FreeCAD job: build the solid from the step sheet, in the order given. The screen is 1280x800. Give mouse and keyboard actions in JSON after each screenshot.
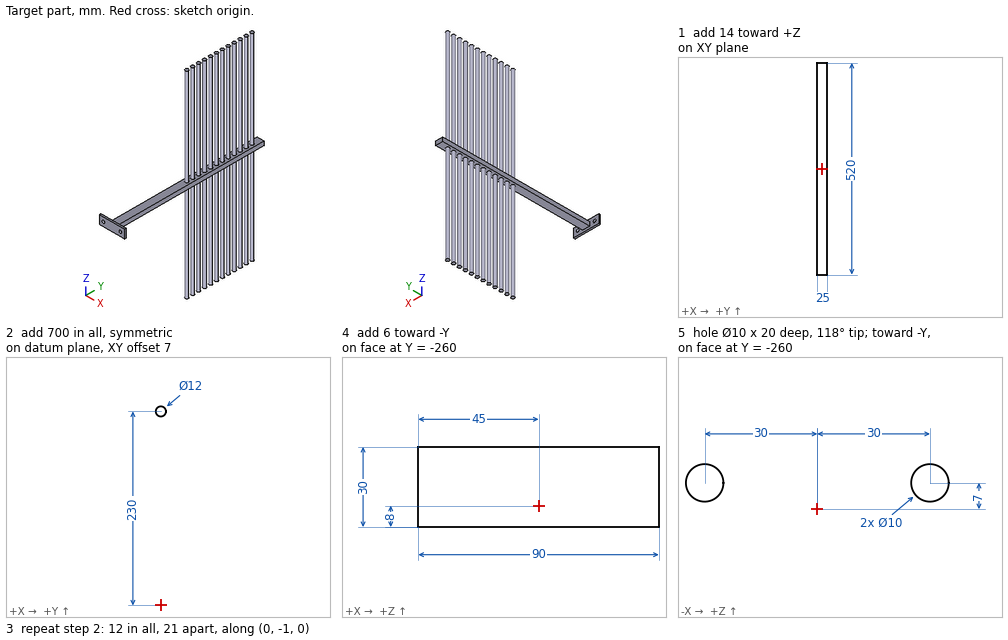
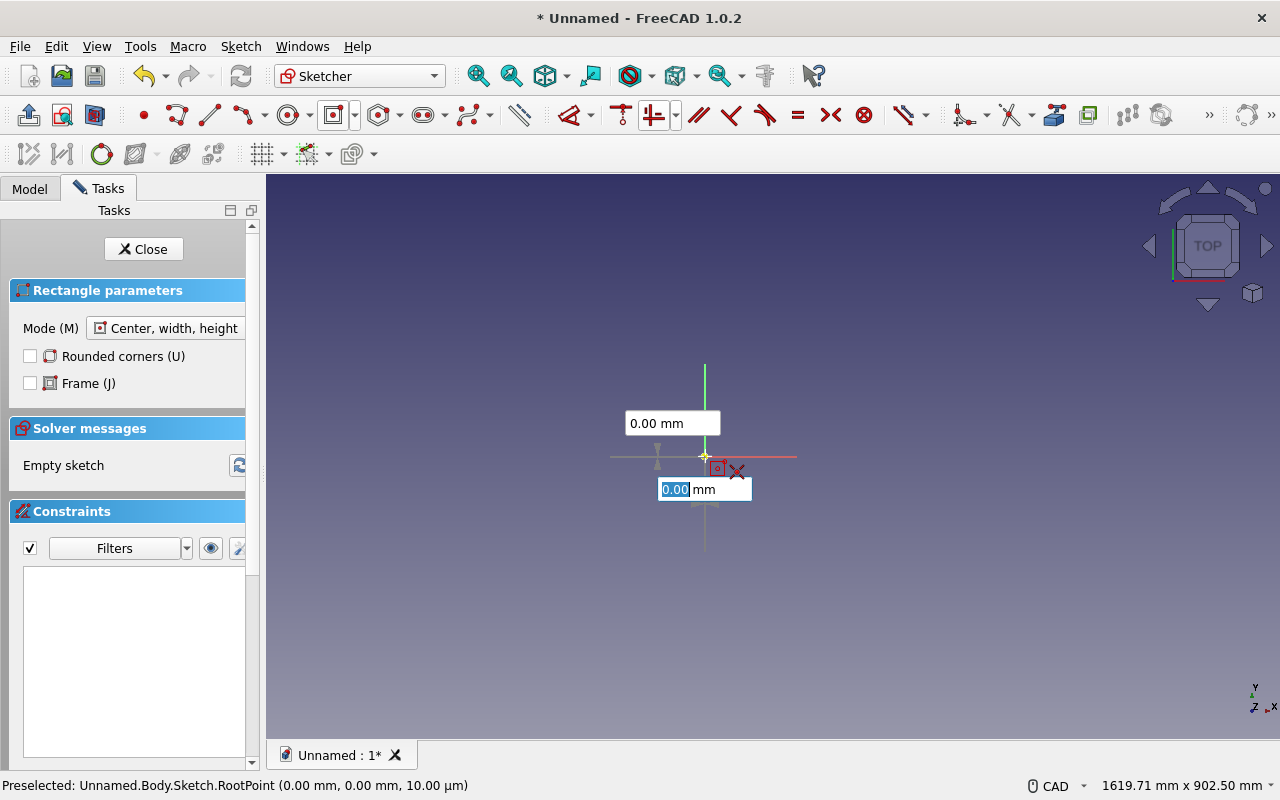
{"action": "scroll", "coordinate": [713, 294], "scroll_direction": "up", "scroll_amount": 4}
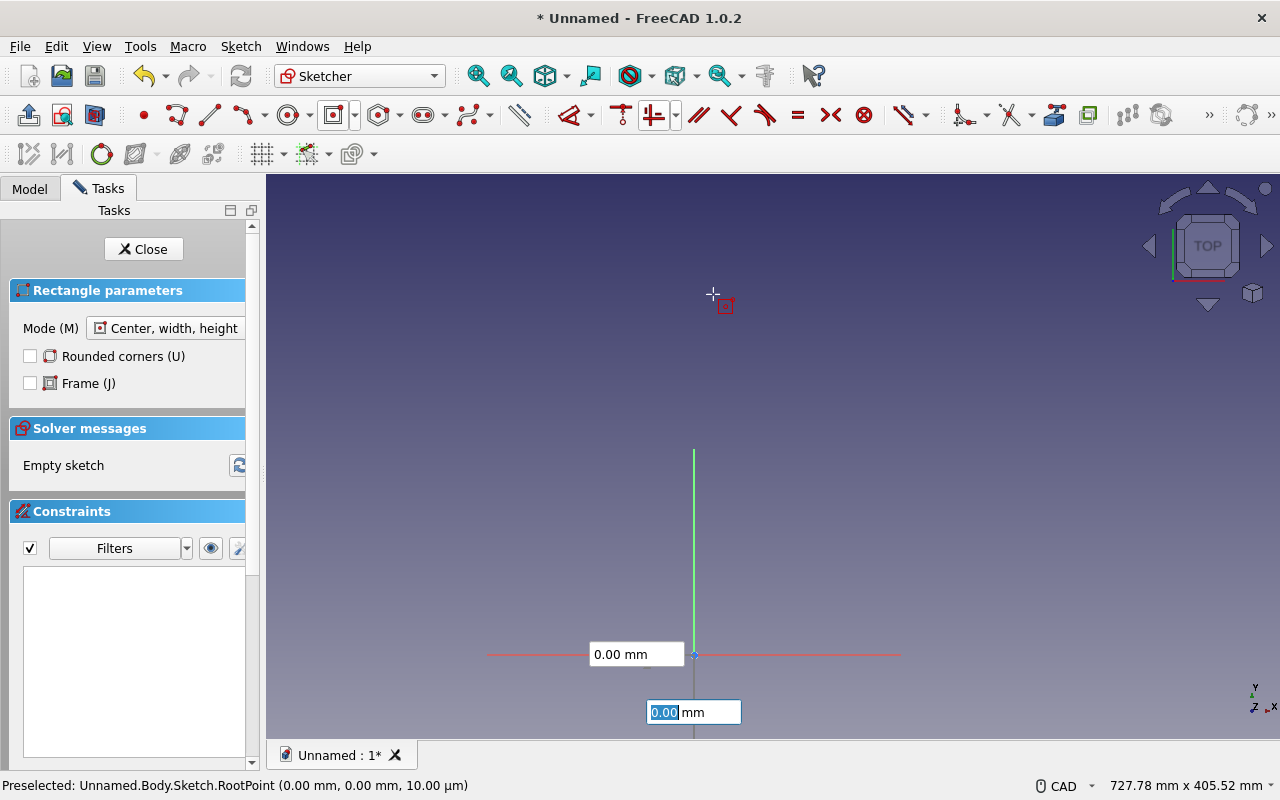
{"action": "left_click", "coordinate": [712, 293]}
{"action": "key", "text": "Escape"}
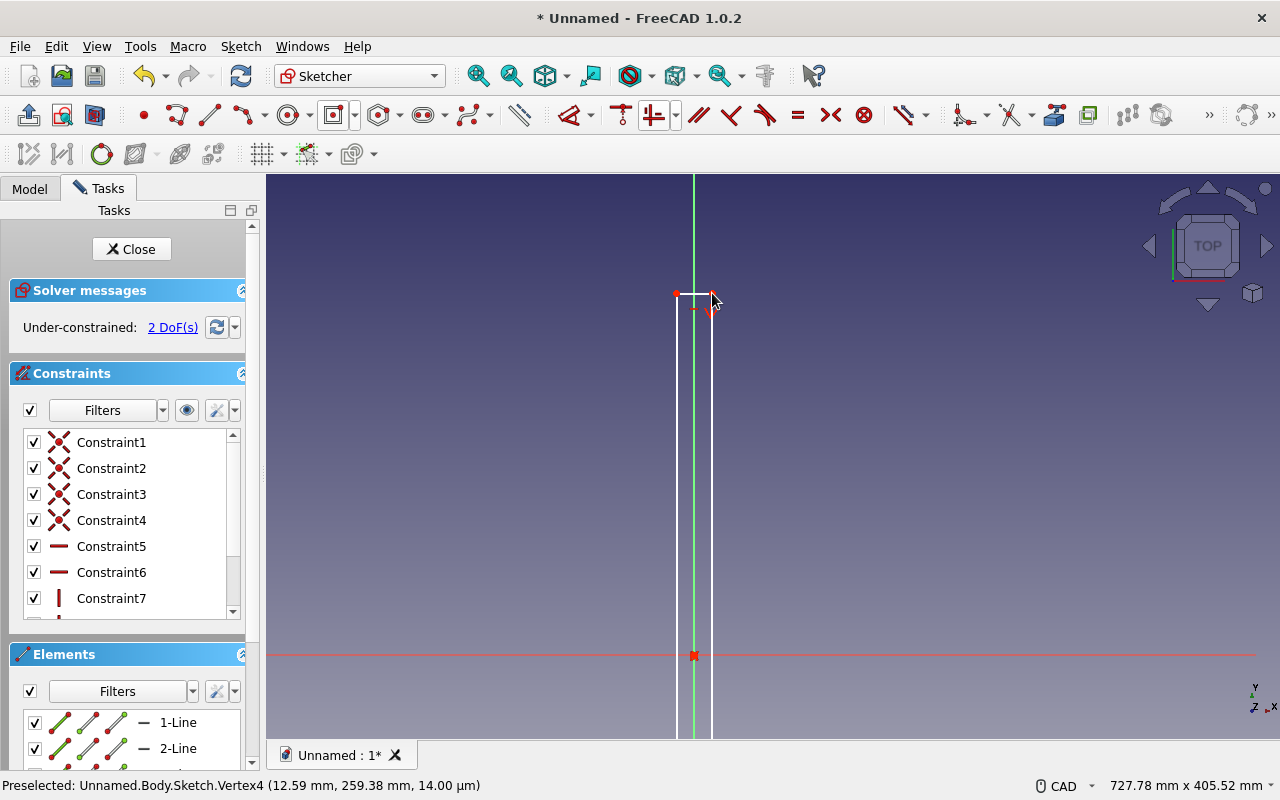
{"action": "left_click", "coordinate": [568, 116]}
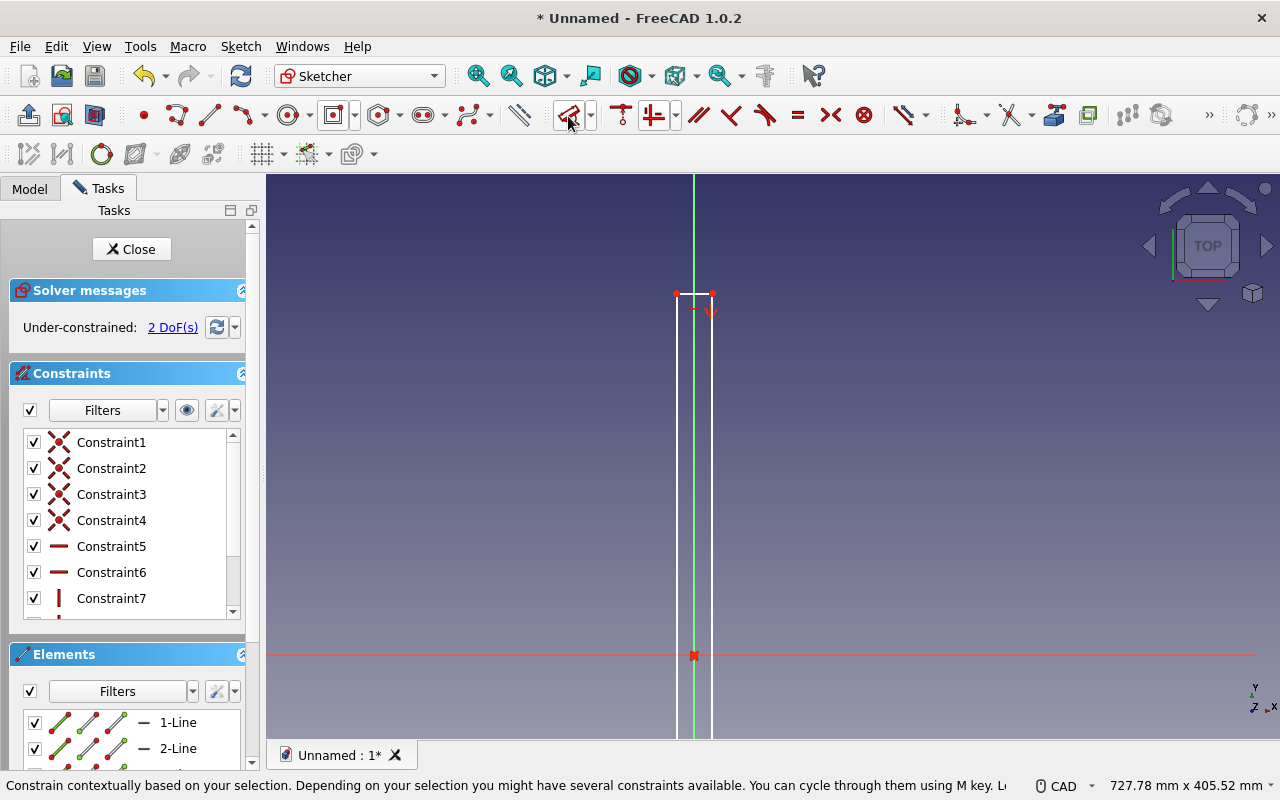
{"action": "scroll", "coordinate": [713, 294], "scroll_direction": "down", "scroll_amount": 4}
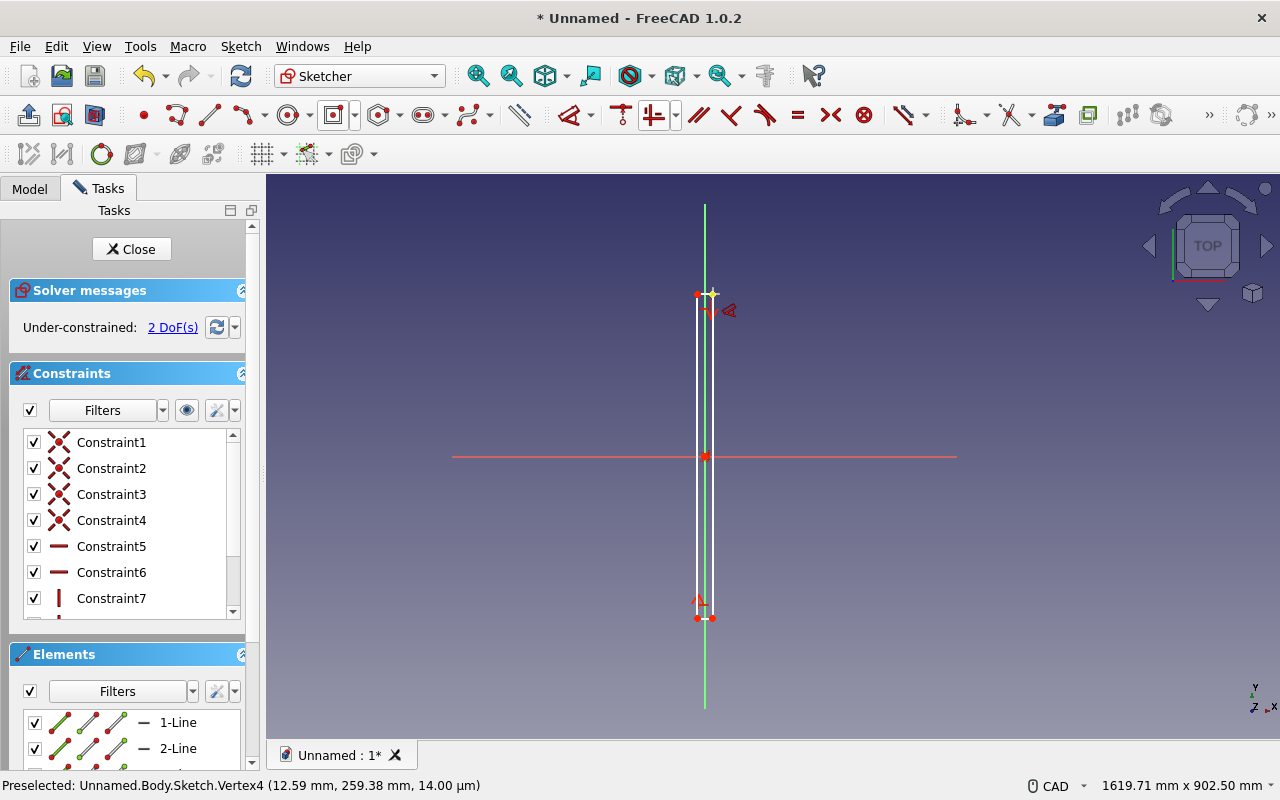
{"action": "scroll", "coordinate": [703, 619], "scroll_direction": "up", "scroll_amount": 5}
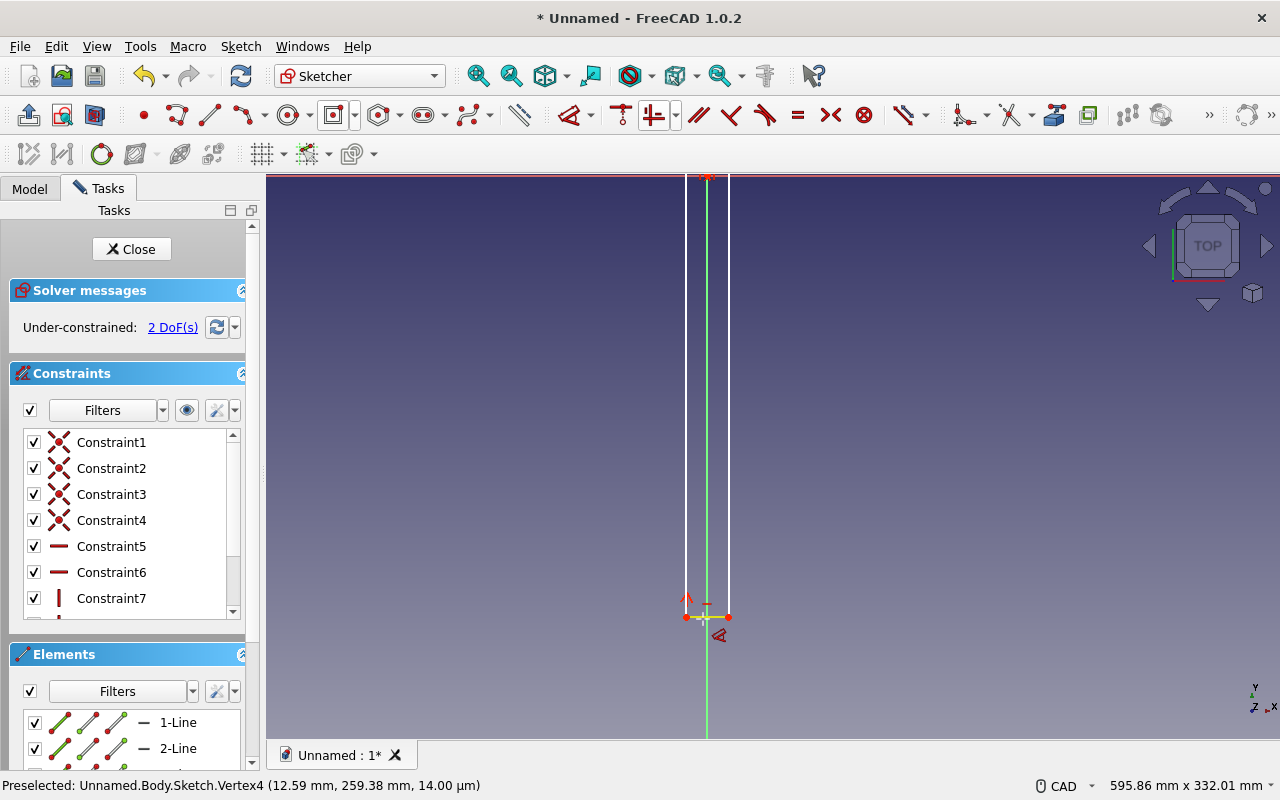
{"action": "left_click", "coordinate": [703, 617]}
{"action": "left_click", "coordinate": [692, 651]}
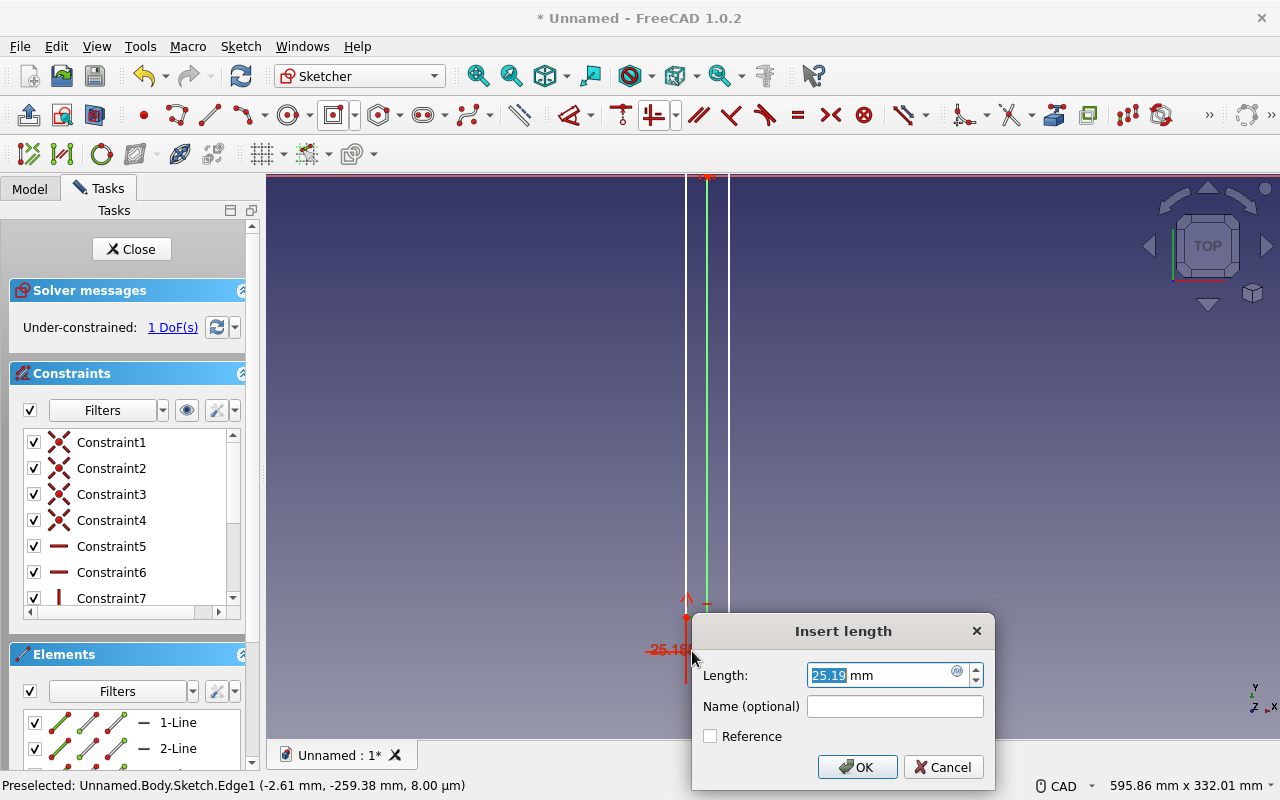
{"action": "type", "text": "25"}
{"action": "key", "text": "Return"}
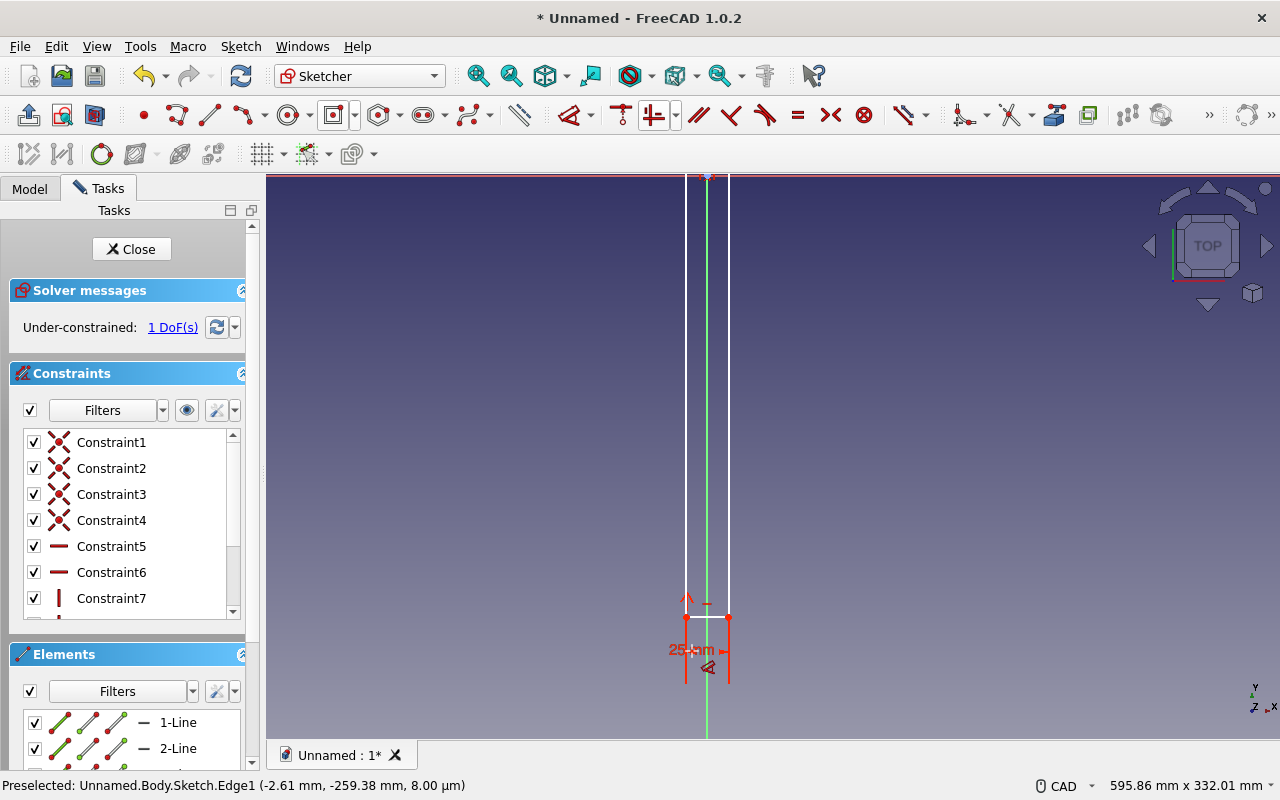
{"action": "left_click", "coordinate": [729, 352]}
{"action": "left_click", "coordinate": [763, 410]}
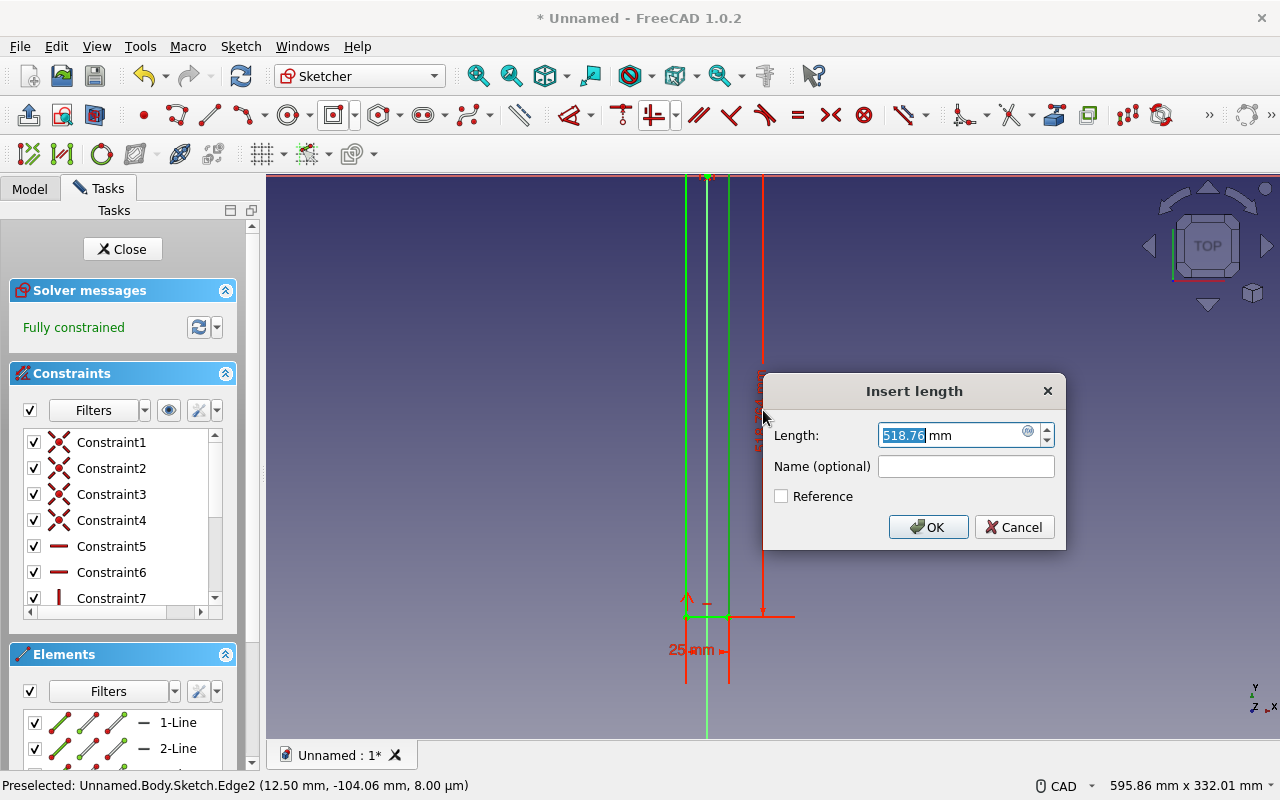
{"action": "type", "text": "520"}
{"action": "key", "text": "Return"}
{"action": "key", "text": "Escape"}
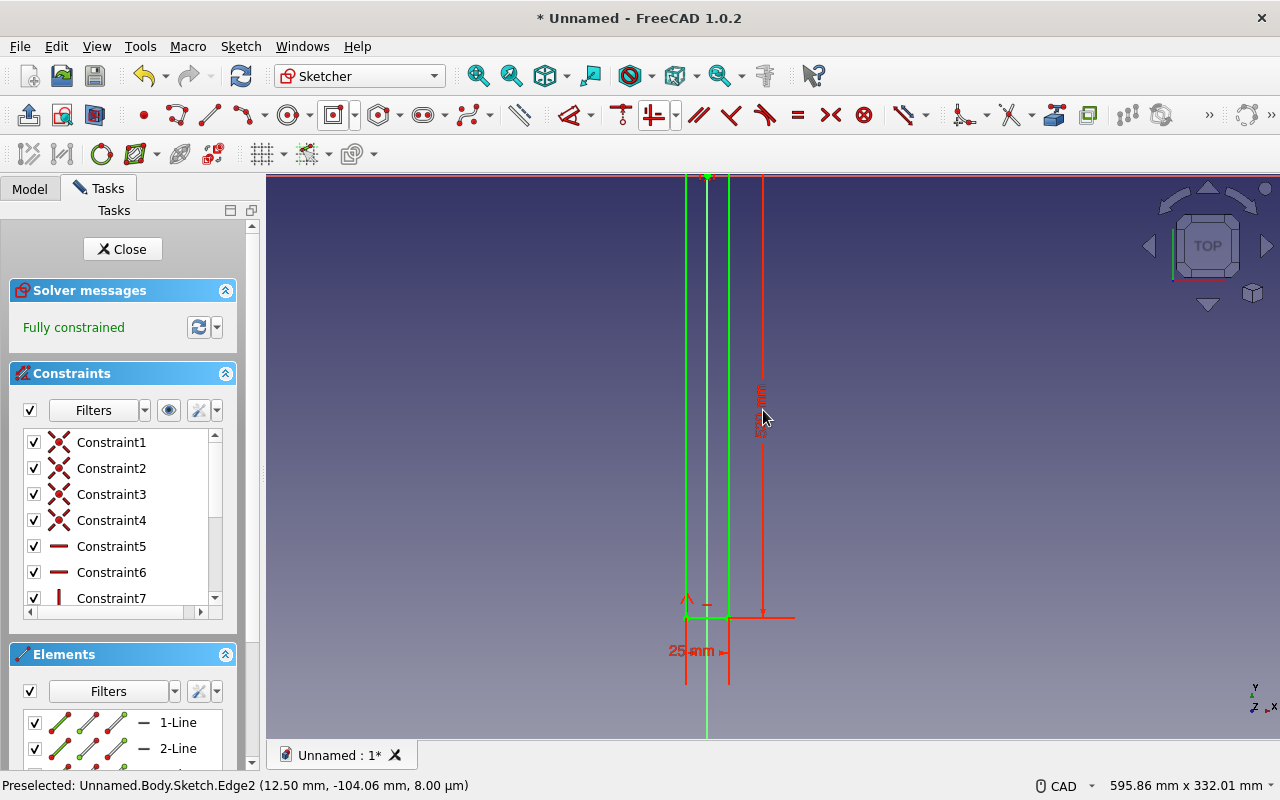
{"action": "left_click", "coordinate": [123, 249]}